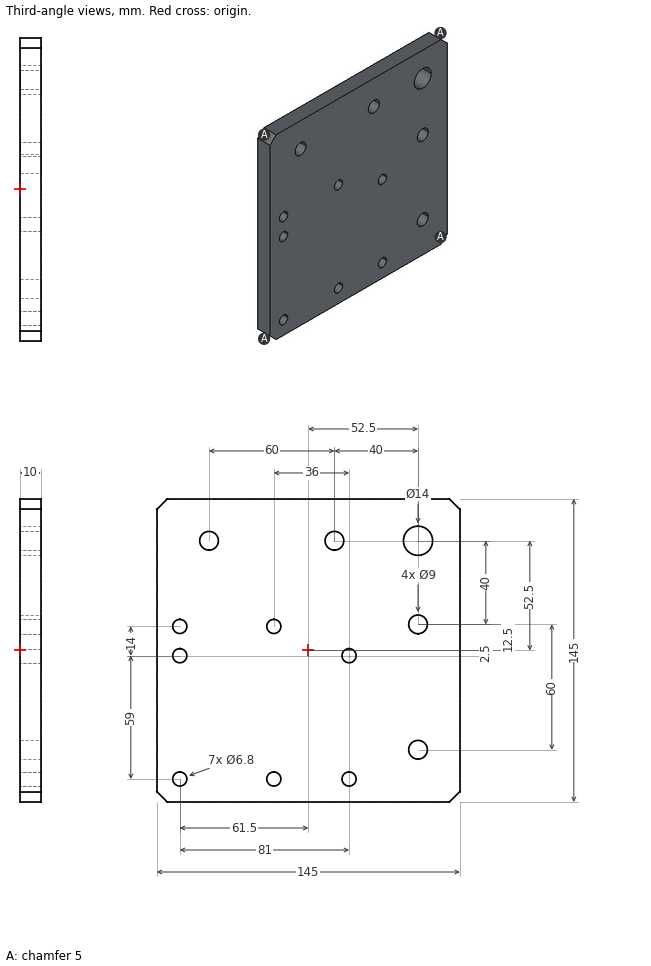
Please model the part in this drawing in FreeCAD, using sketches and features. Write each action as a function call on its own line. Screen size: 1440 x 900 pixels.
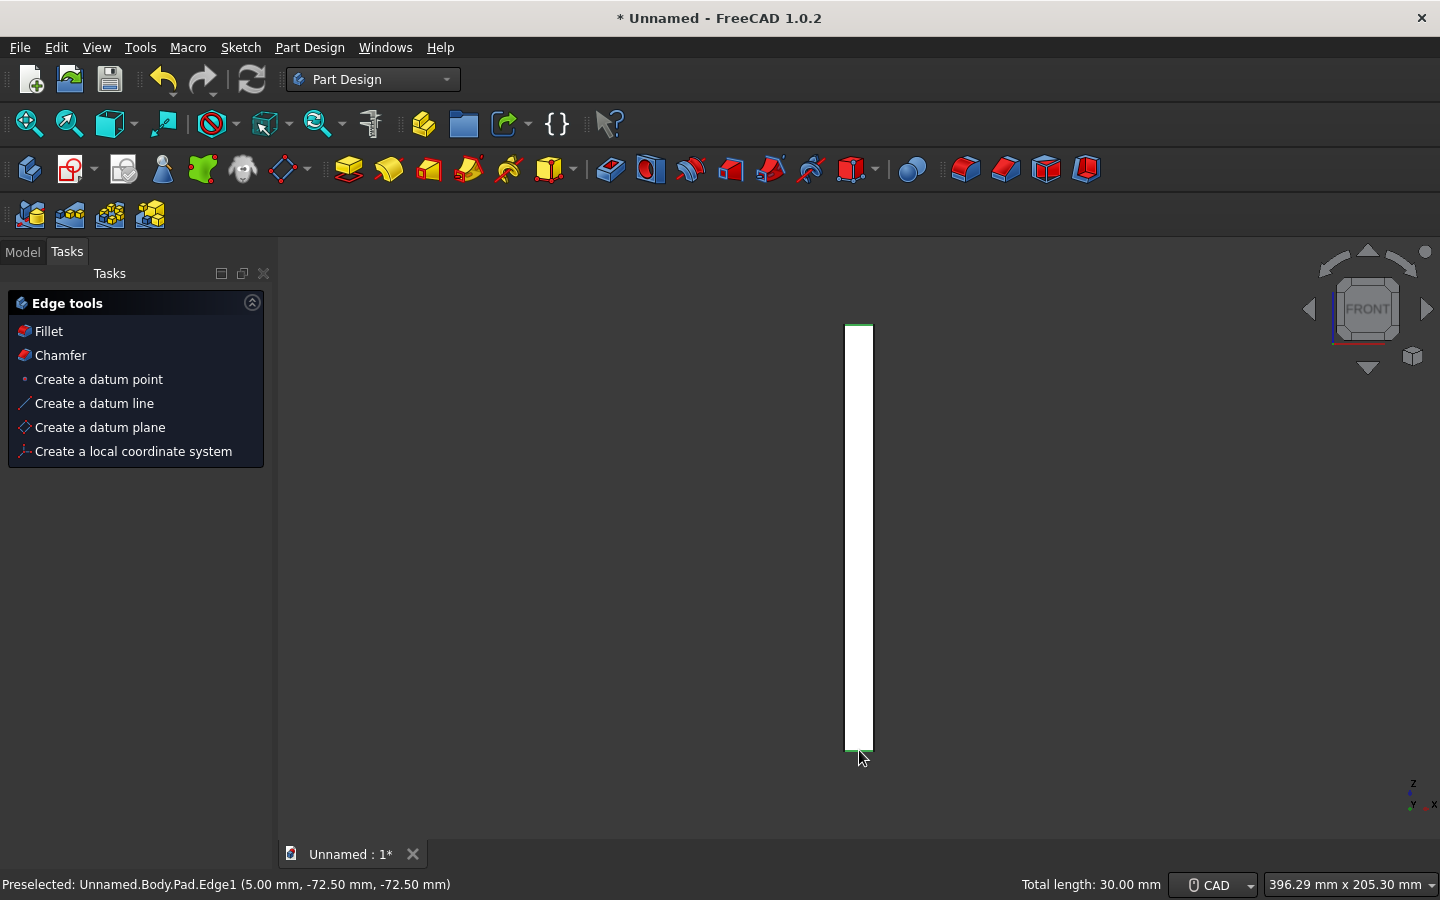
key(3)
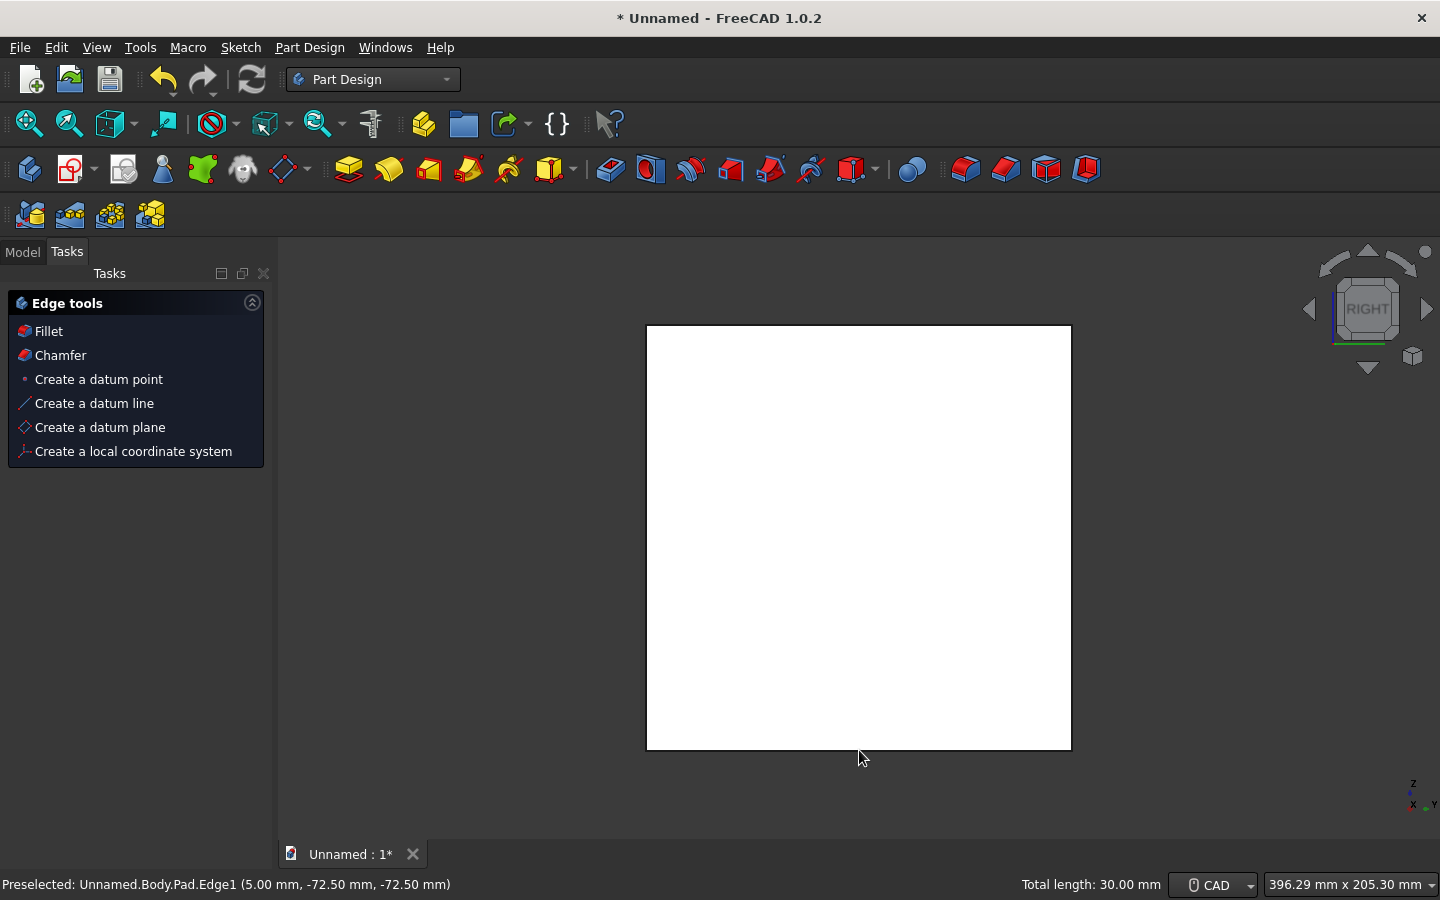
key(5)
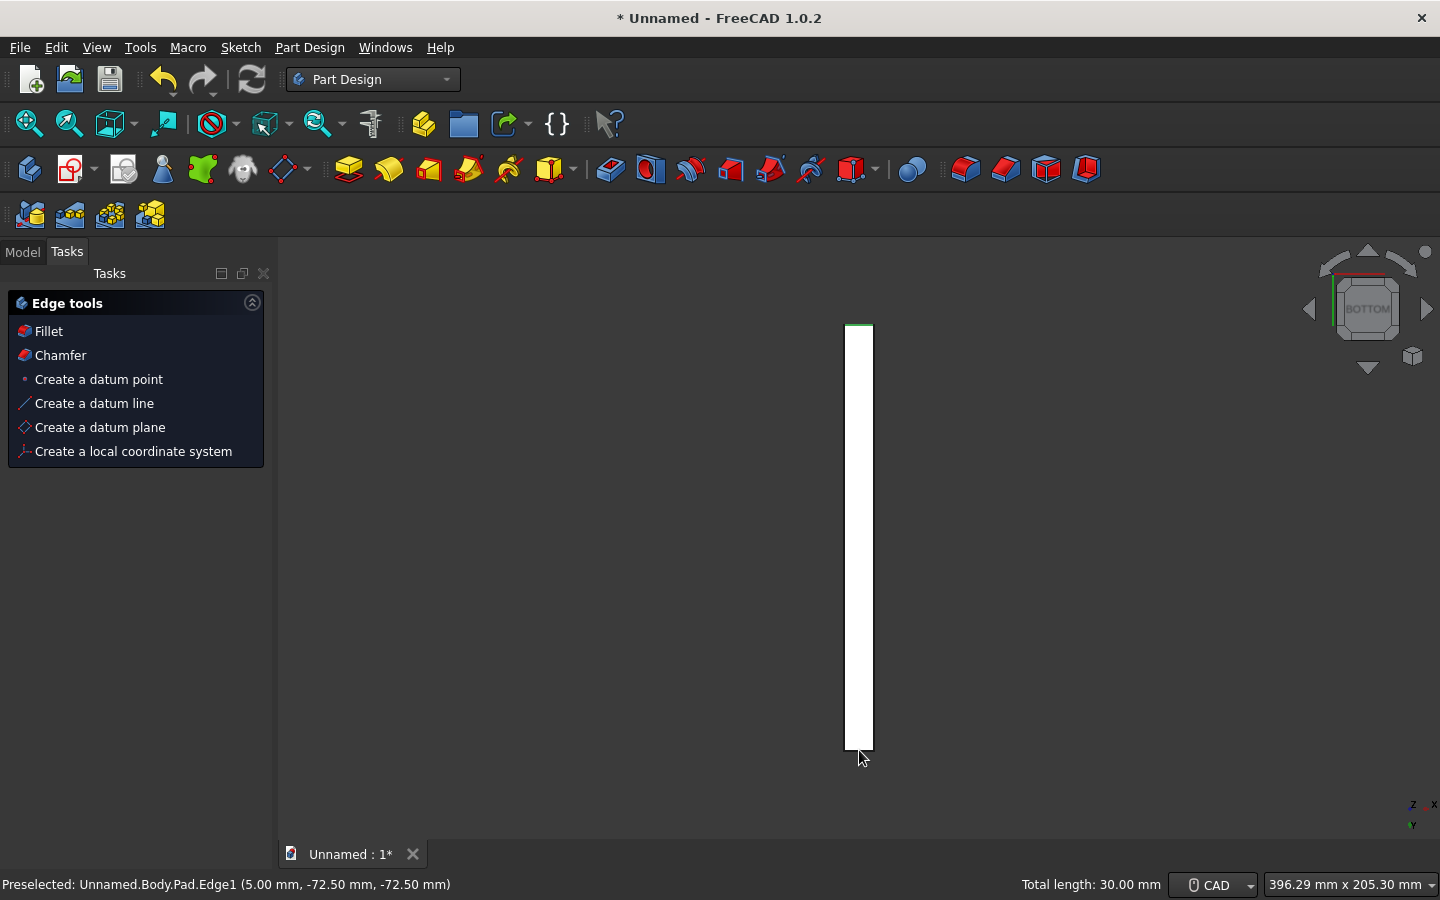
click(859, 750, ctrl)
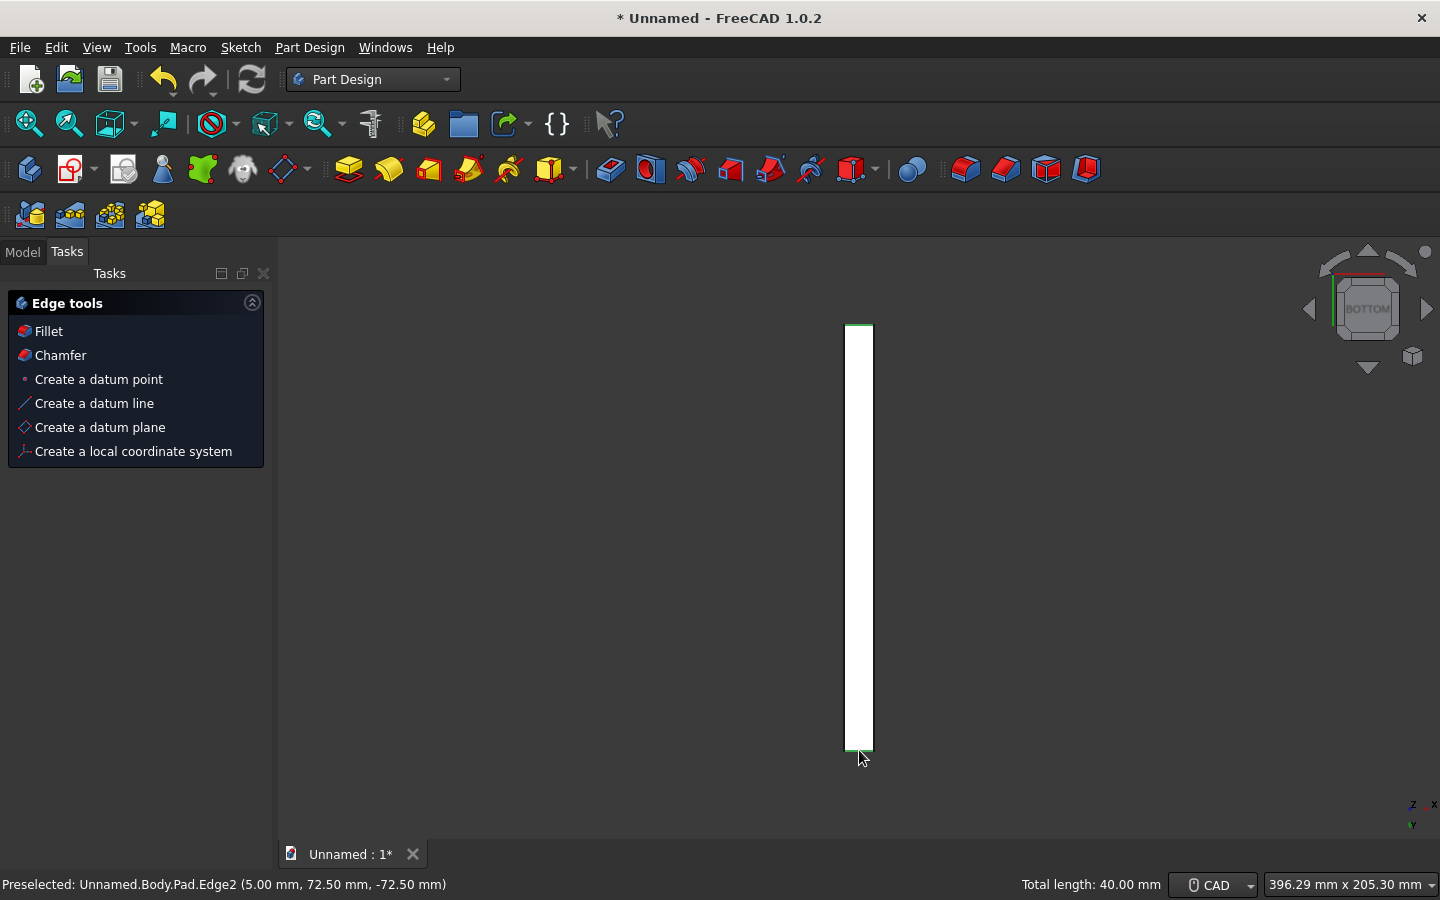
click(1006, 170)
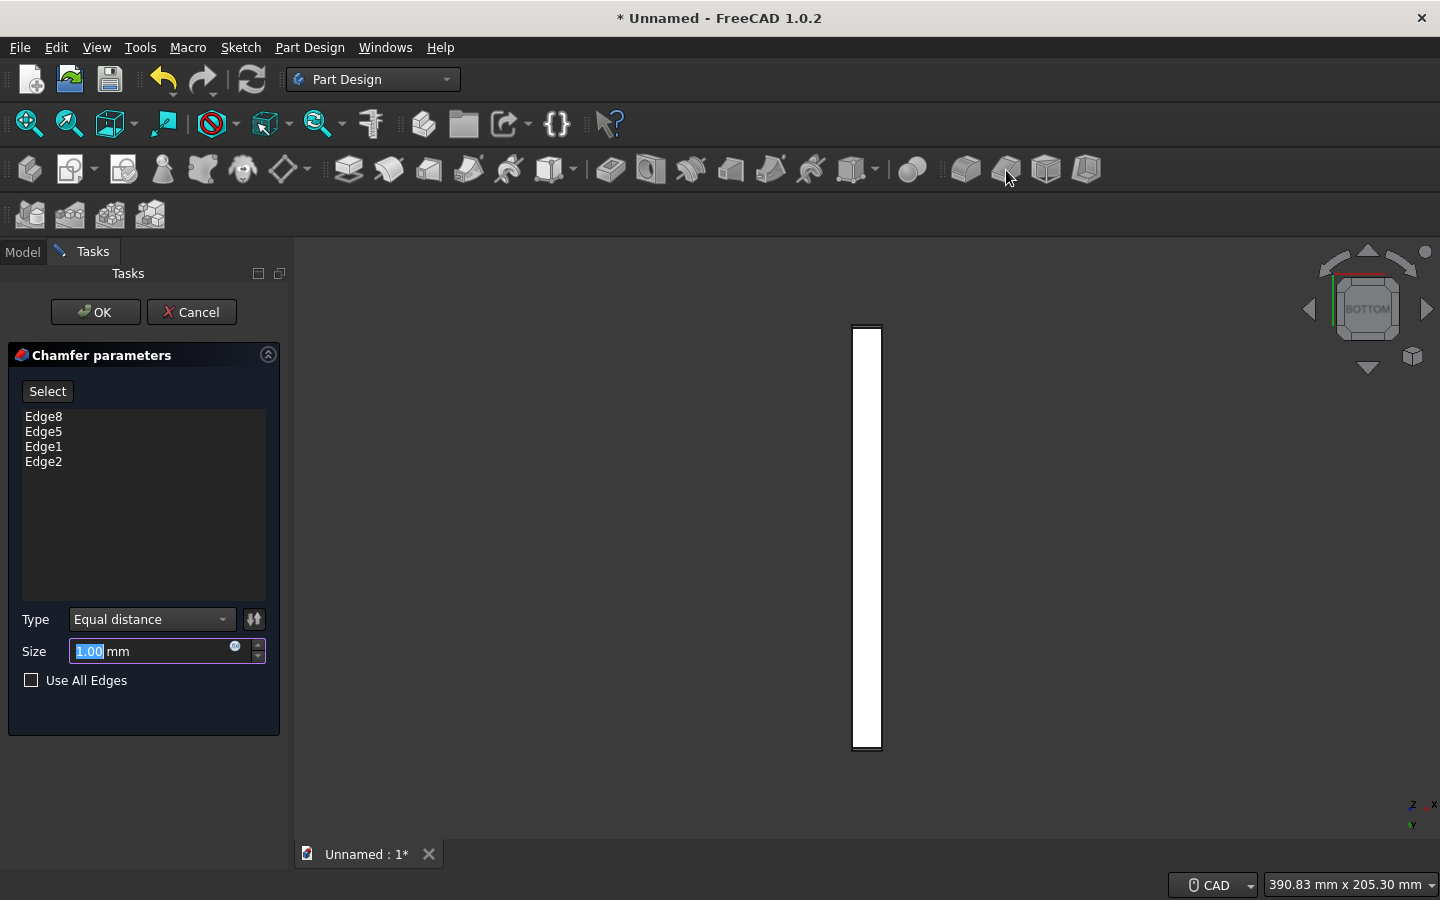
text(5)
key(Tab)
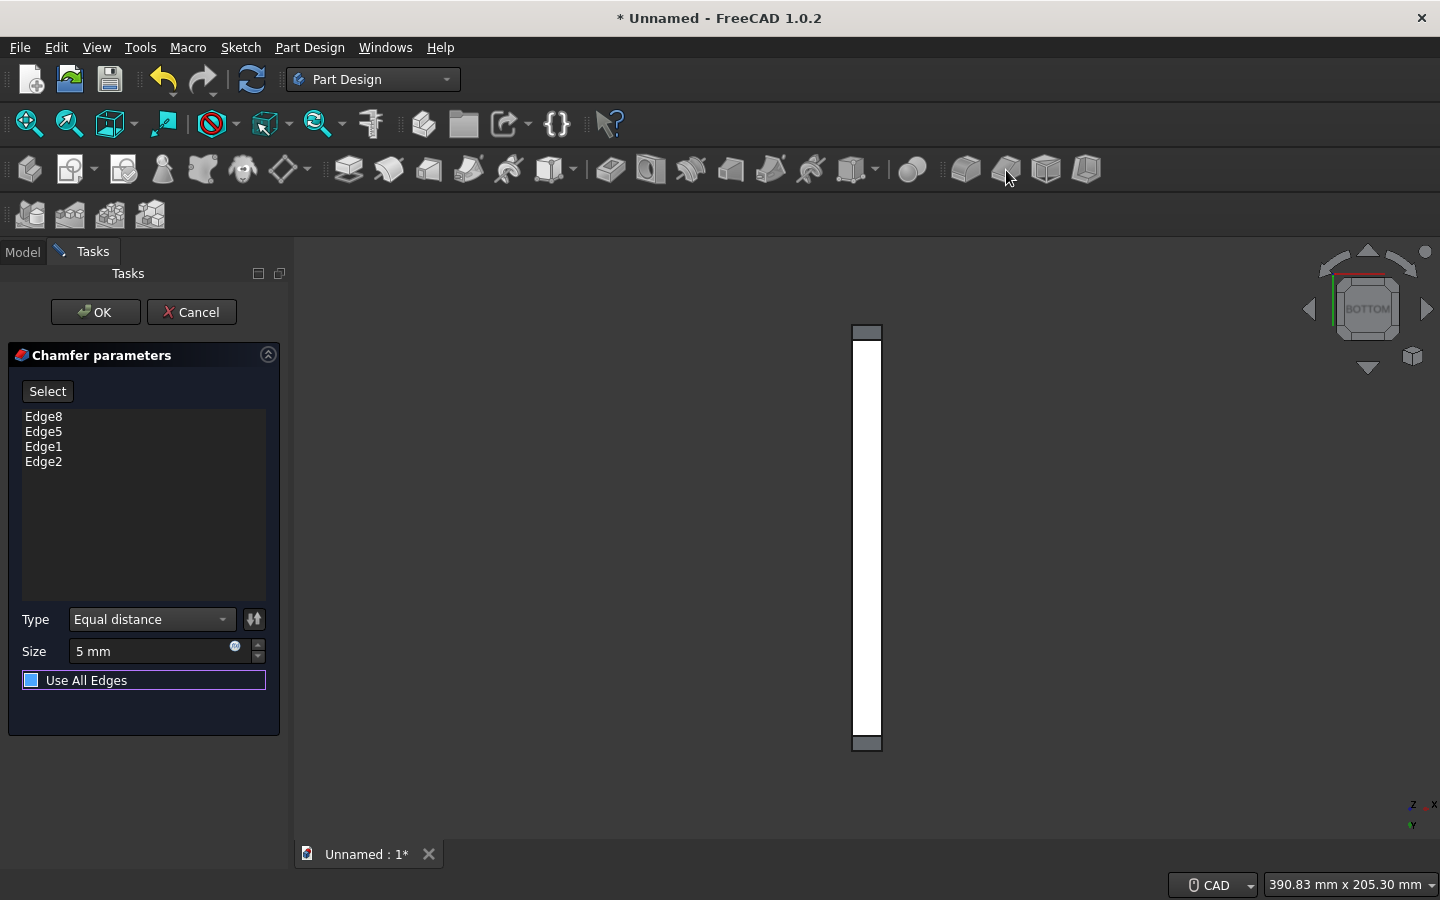
click(96, 312)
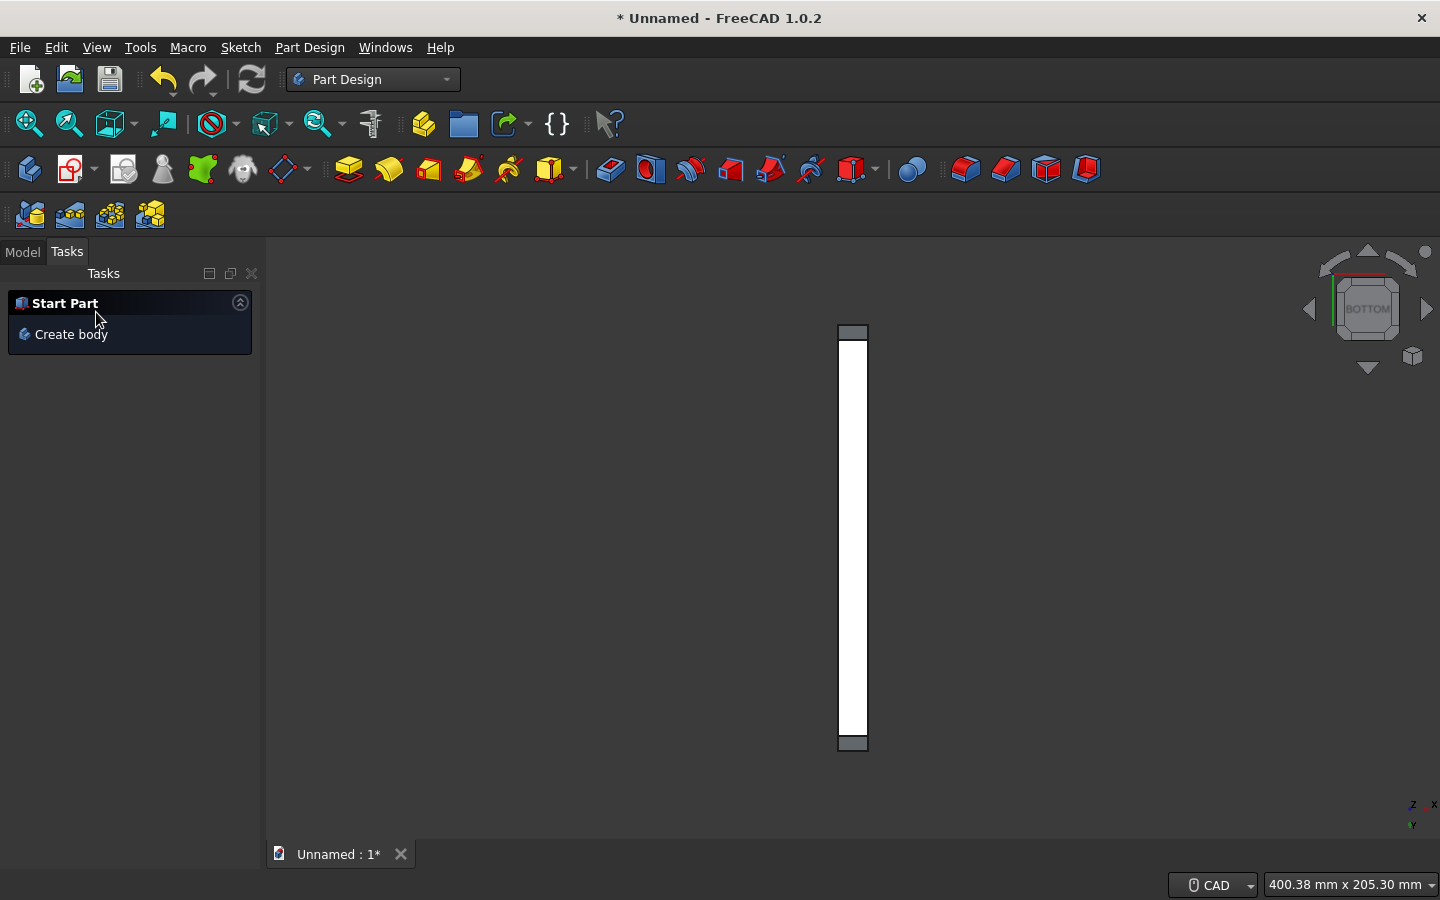
key(0)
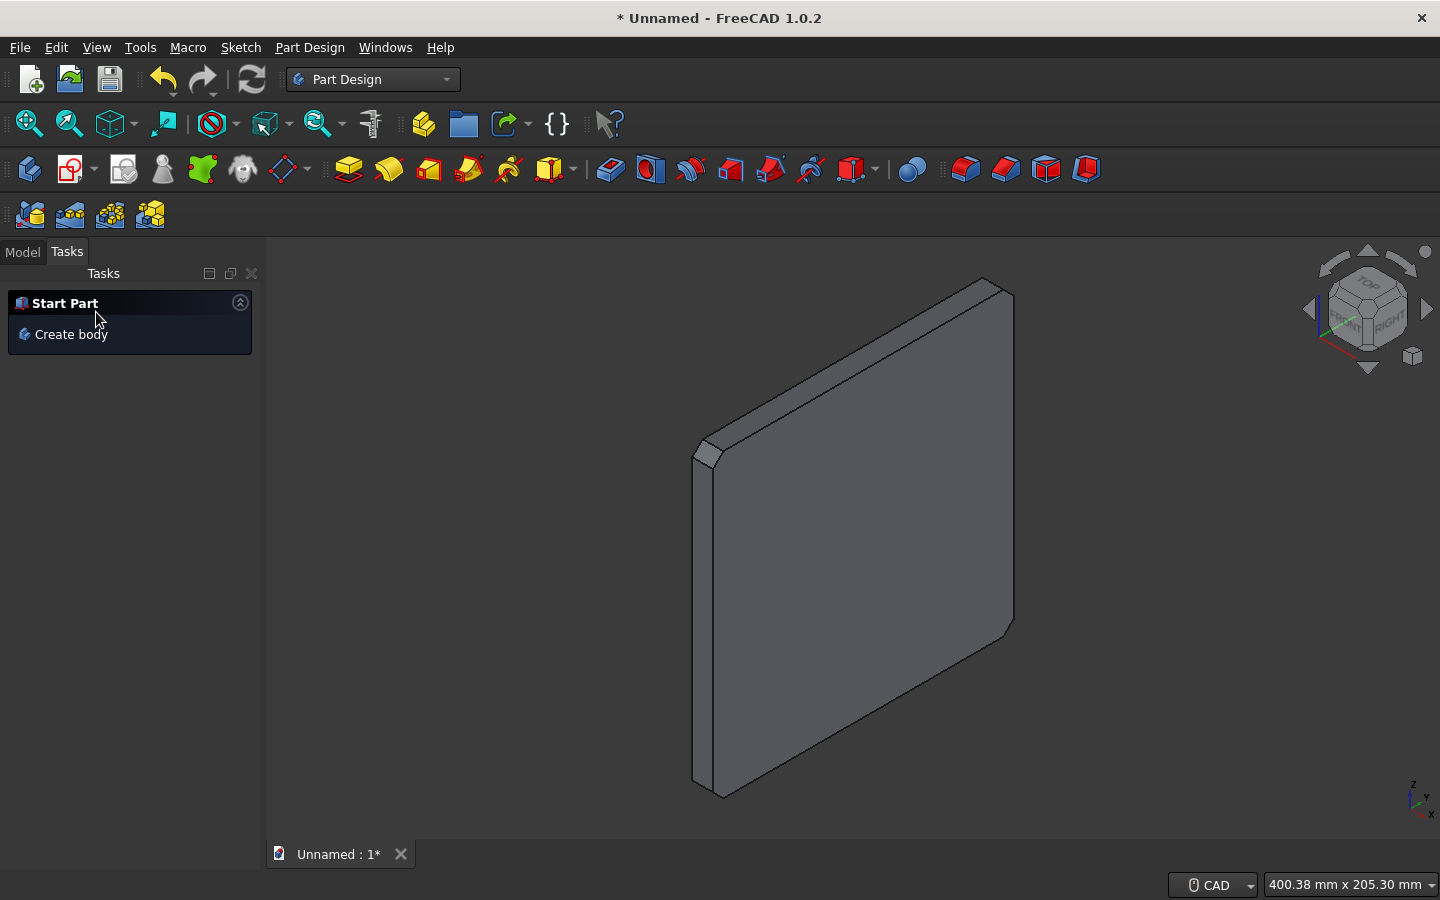
click(863, 543)